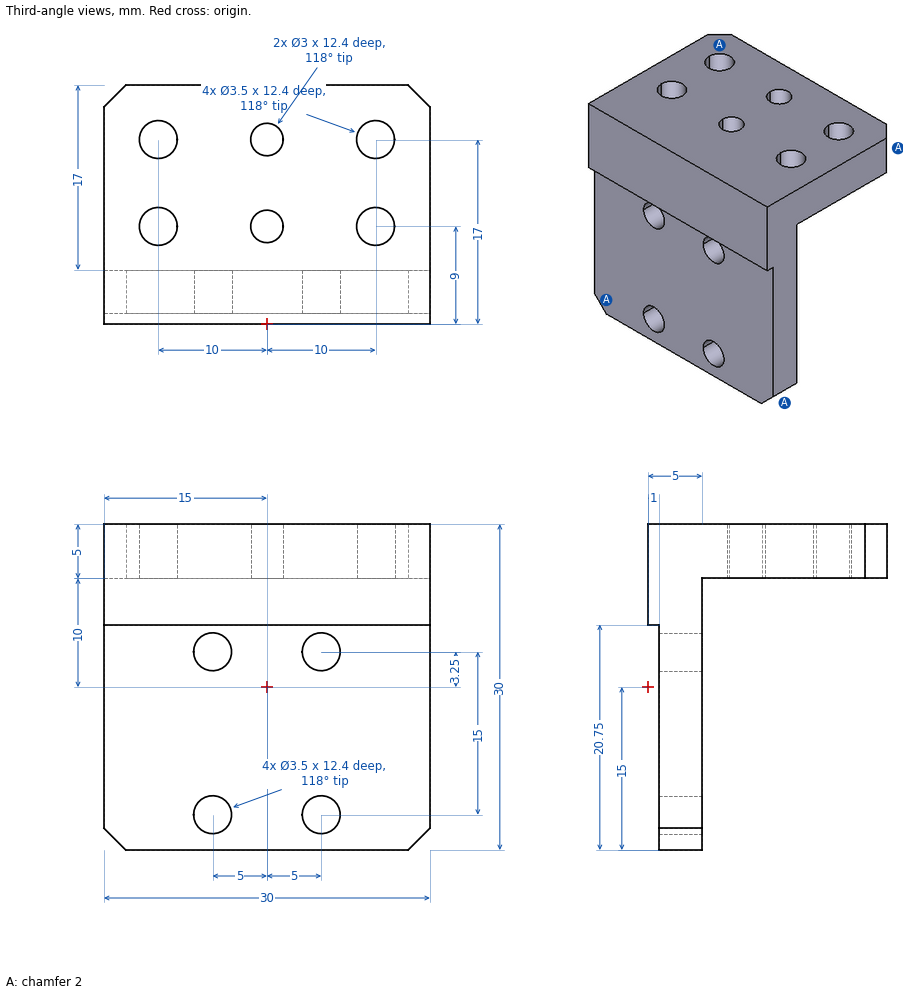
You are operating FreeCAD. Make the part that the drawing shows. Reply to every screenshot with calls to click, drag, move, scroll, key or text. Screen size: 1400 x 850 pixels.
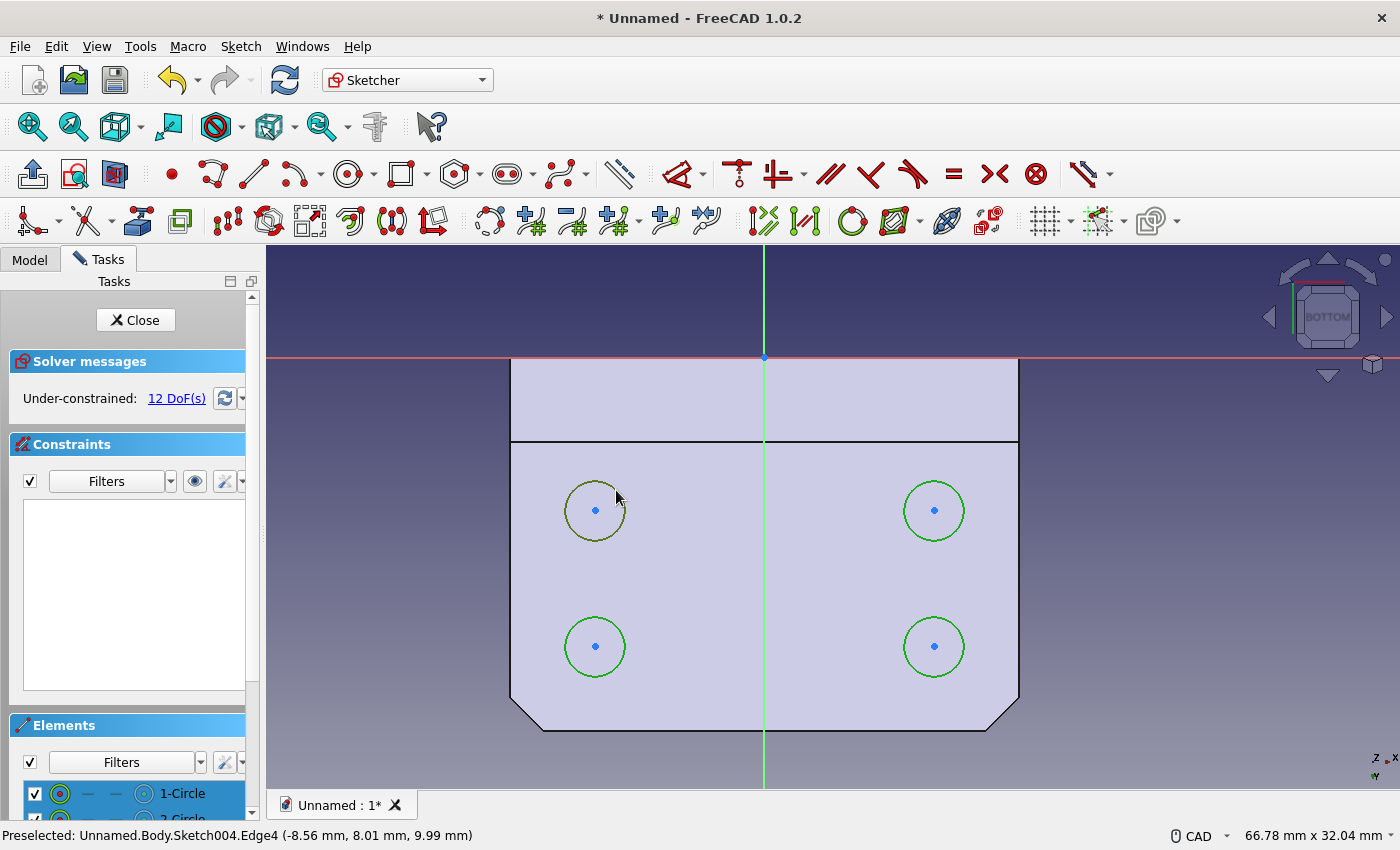
key(e)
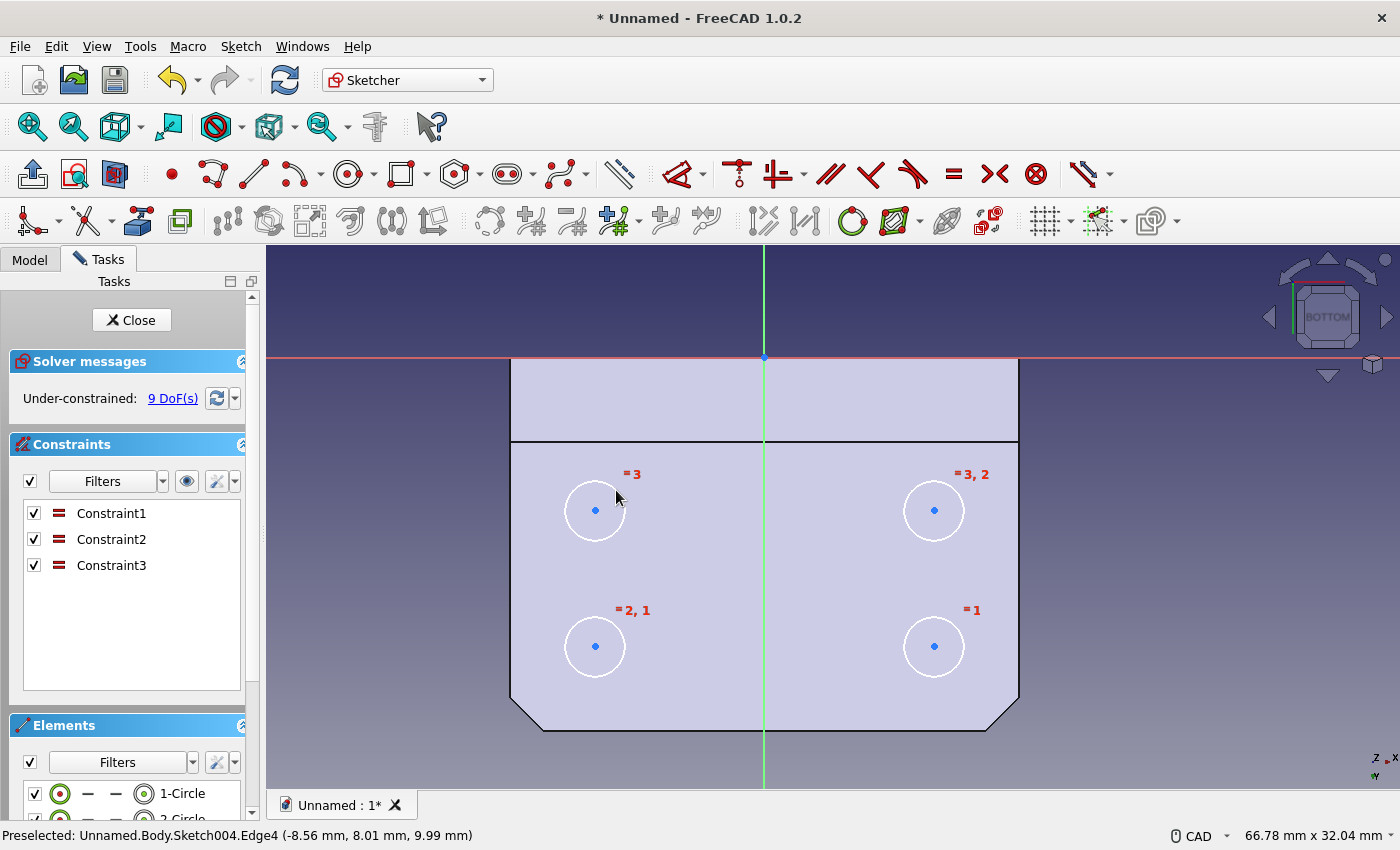
click(934, 647)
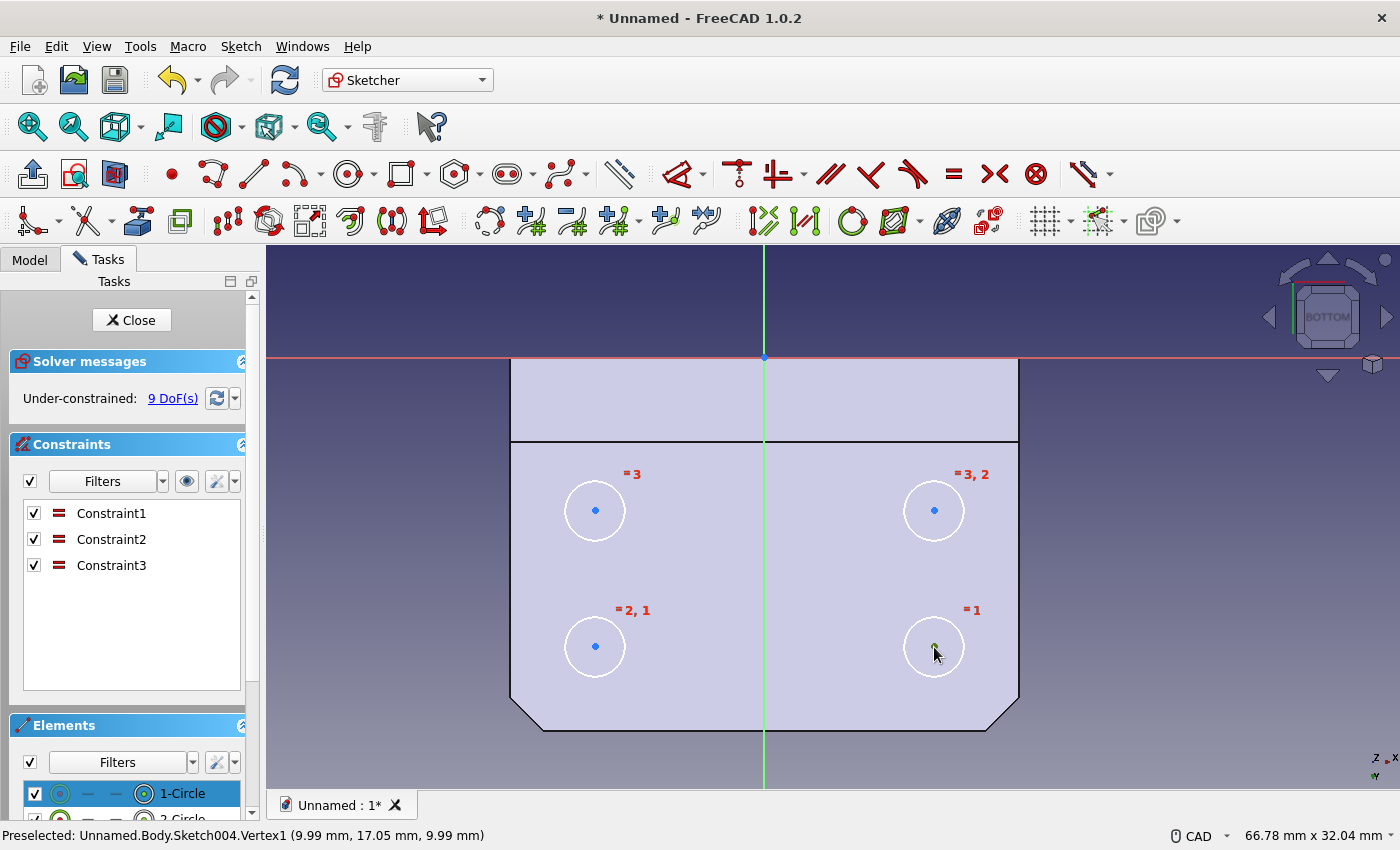
click(595, 647)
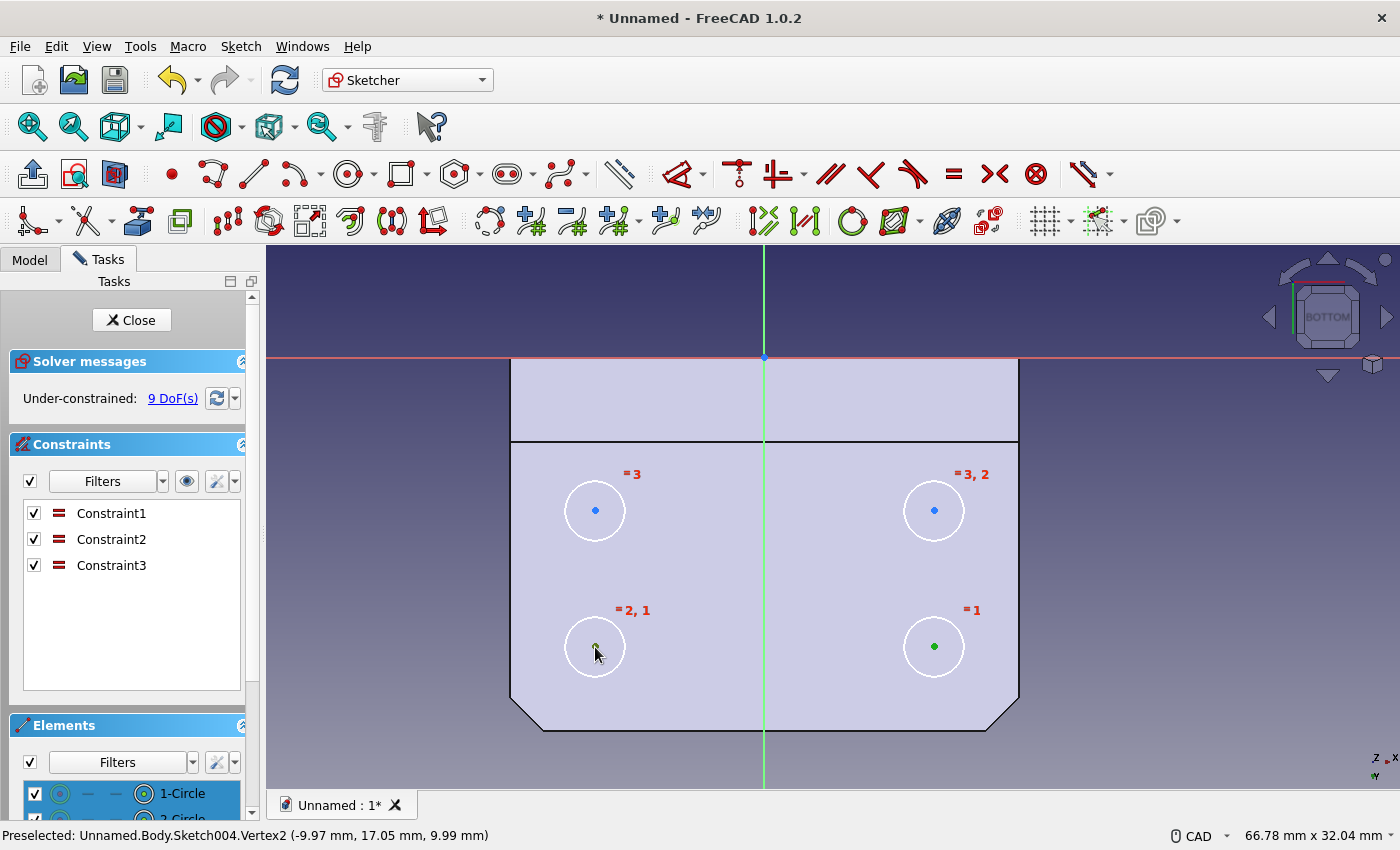
key(h)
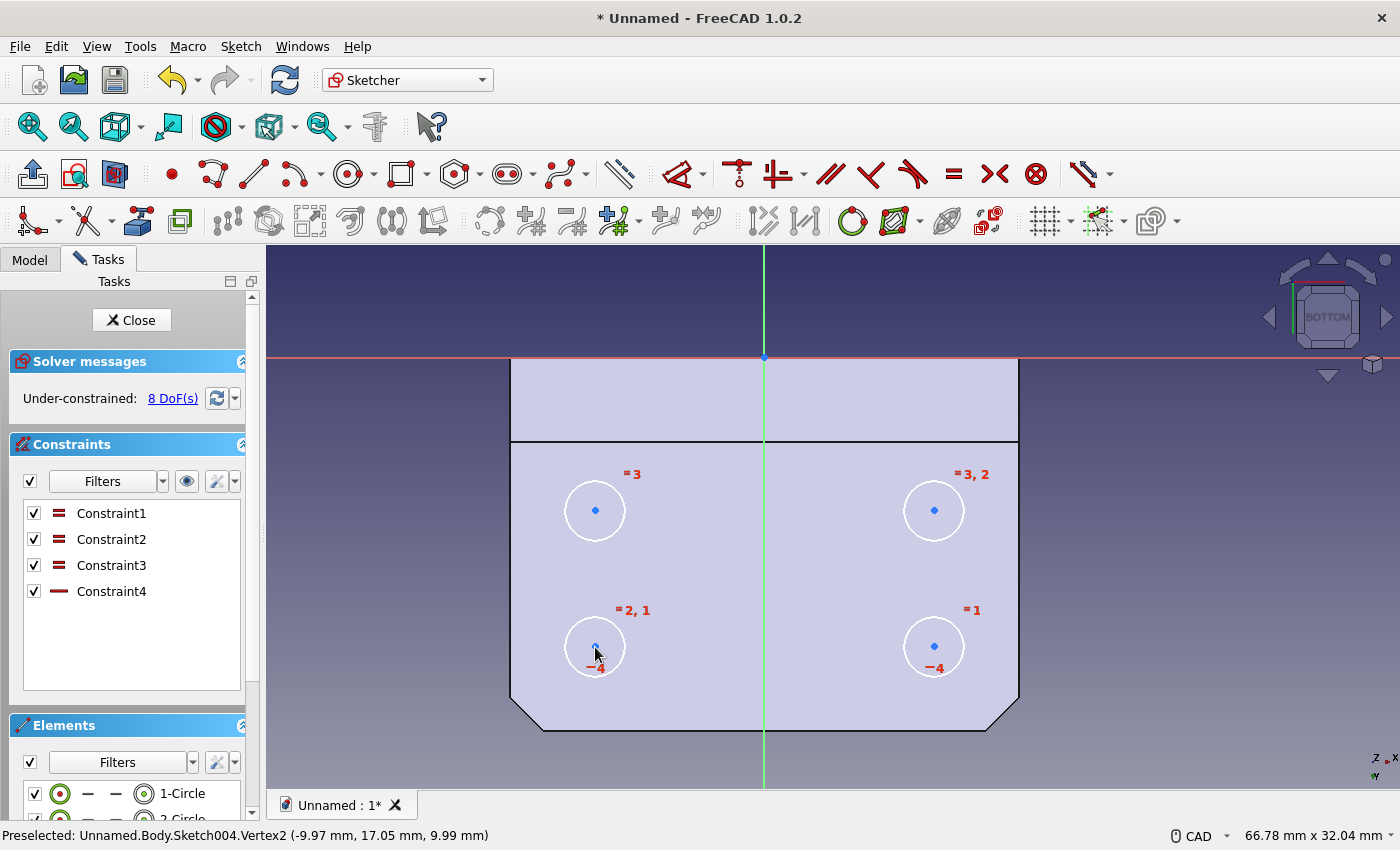
click(934, 647)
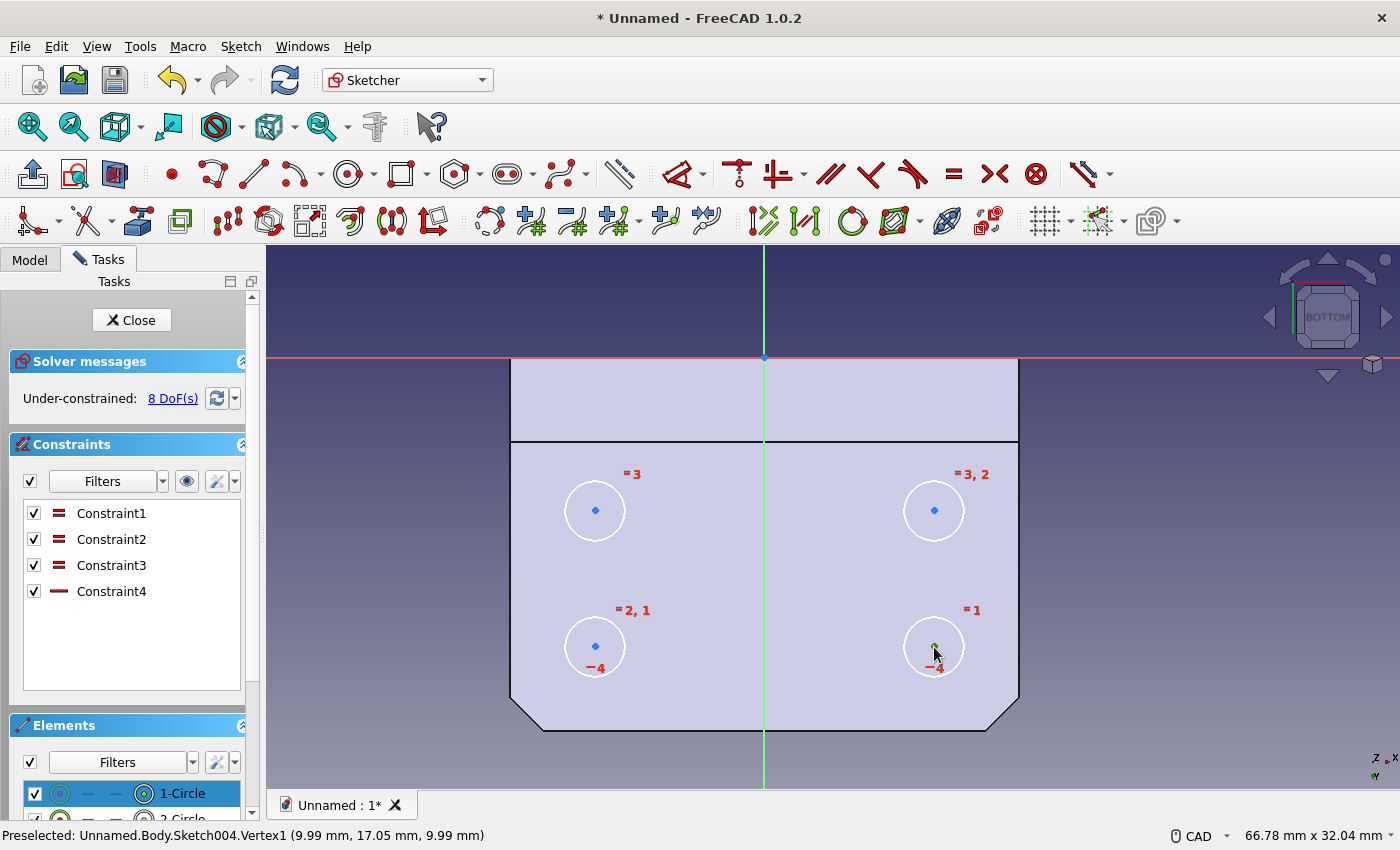
click(934, 511)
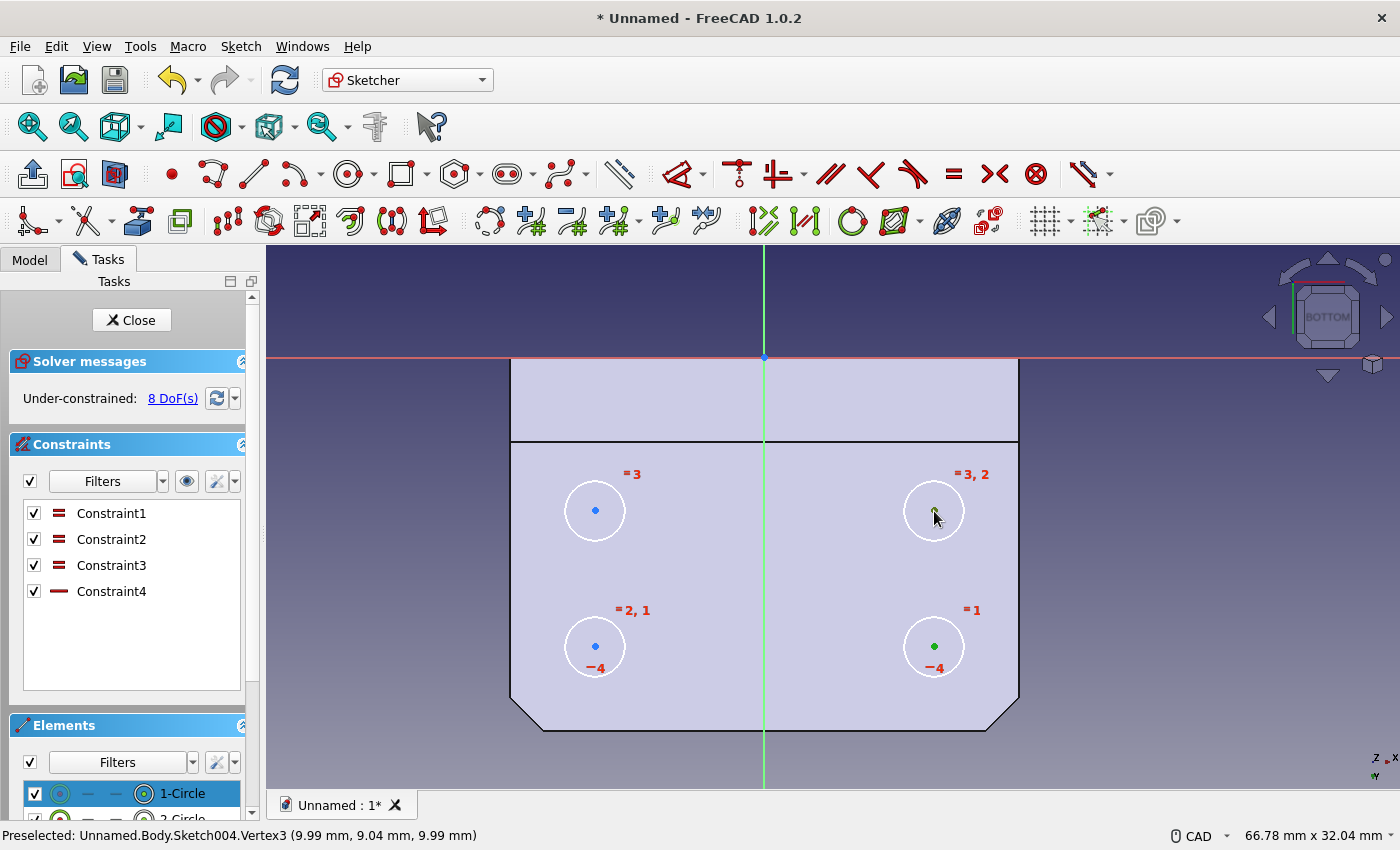
click(804, 174)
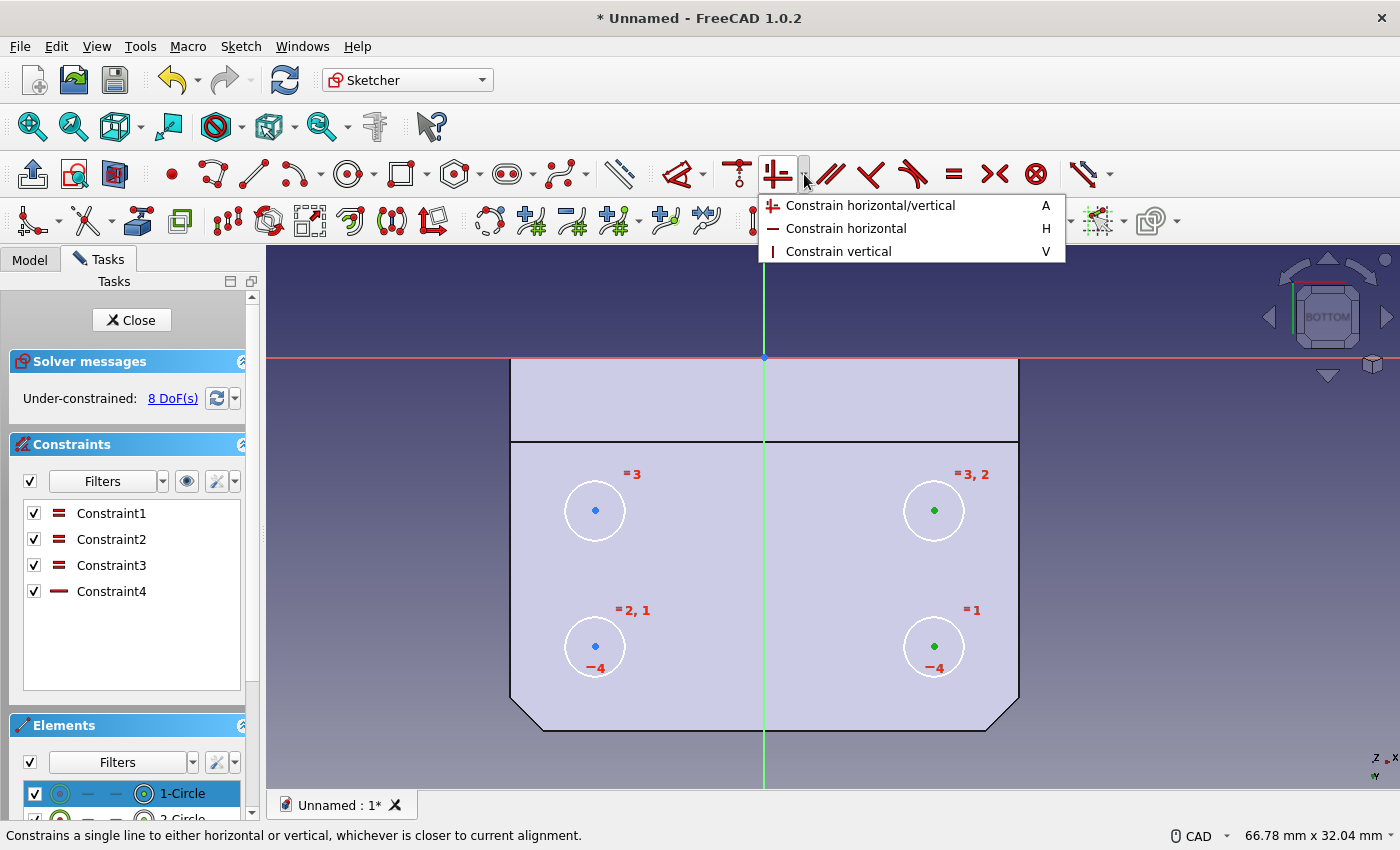
click(912, 252)